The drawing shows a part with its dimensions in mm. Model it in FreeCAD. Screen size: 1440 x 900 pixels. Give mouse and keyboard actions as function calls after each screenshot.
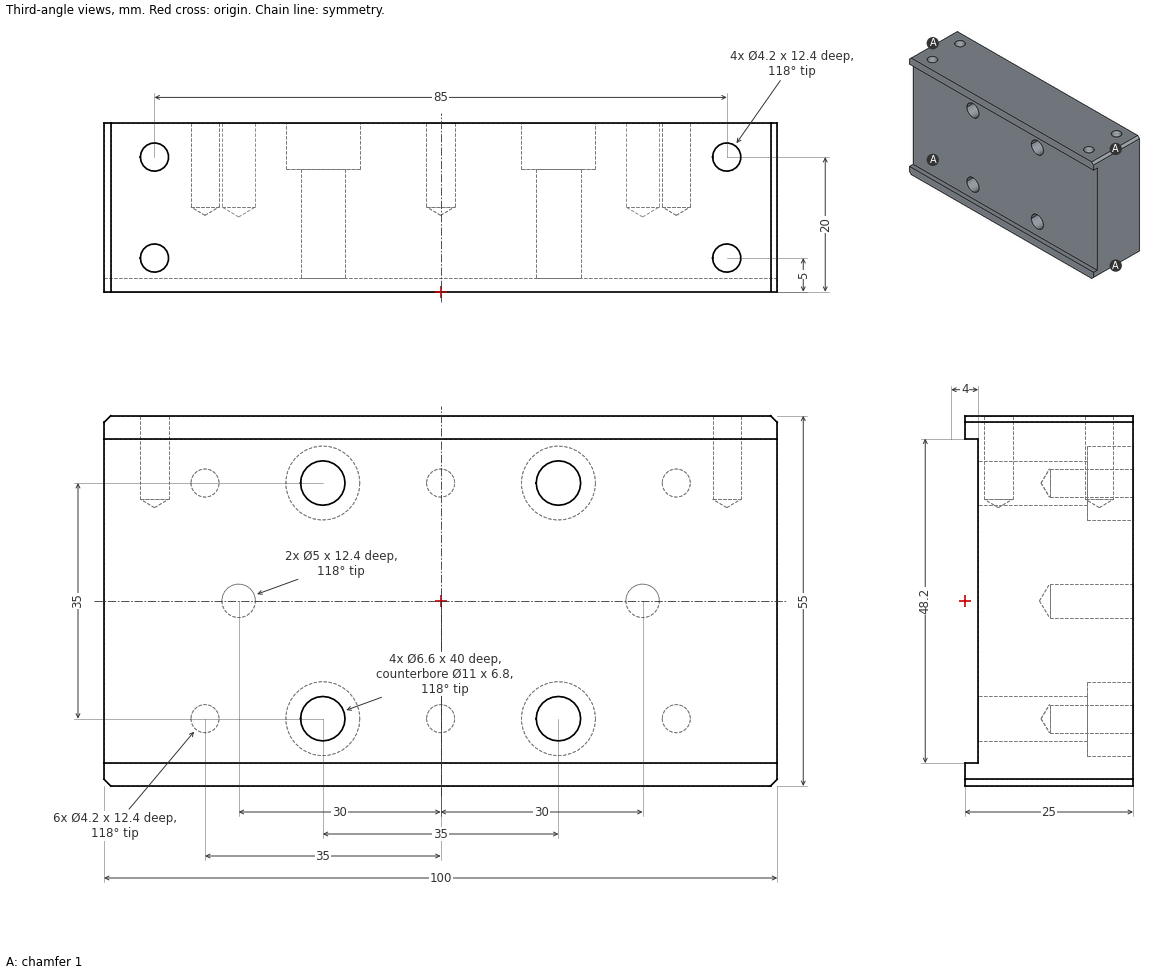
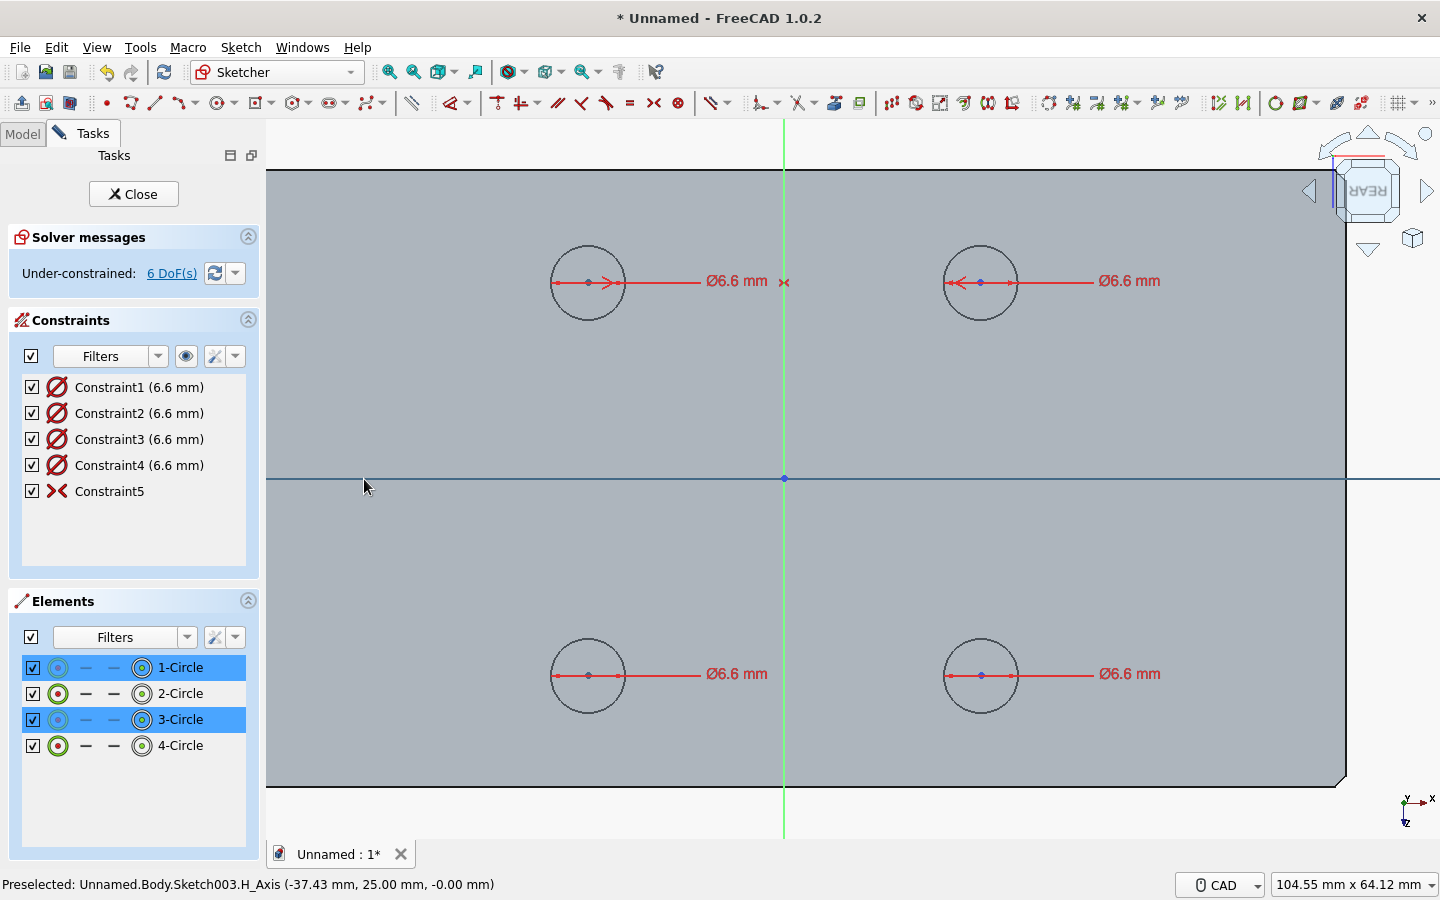
click(654, 104)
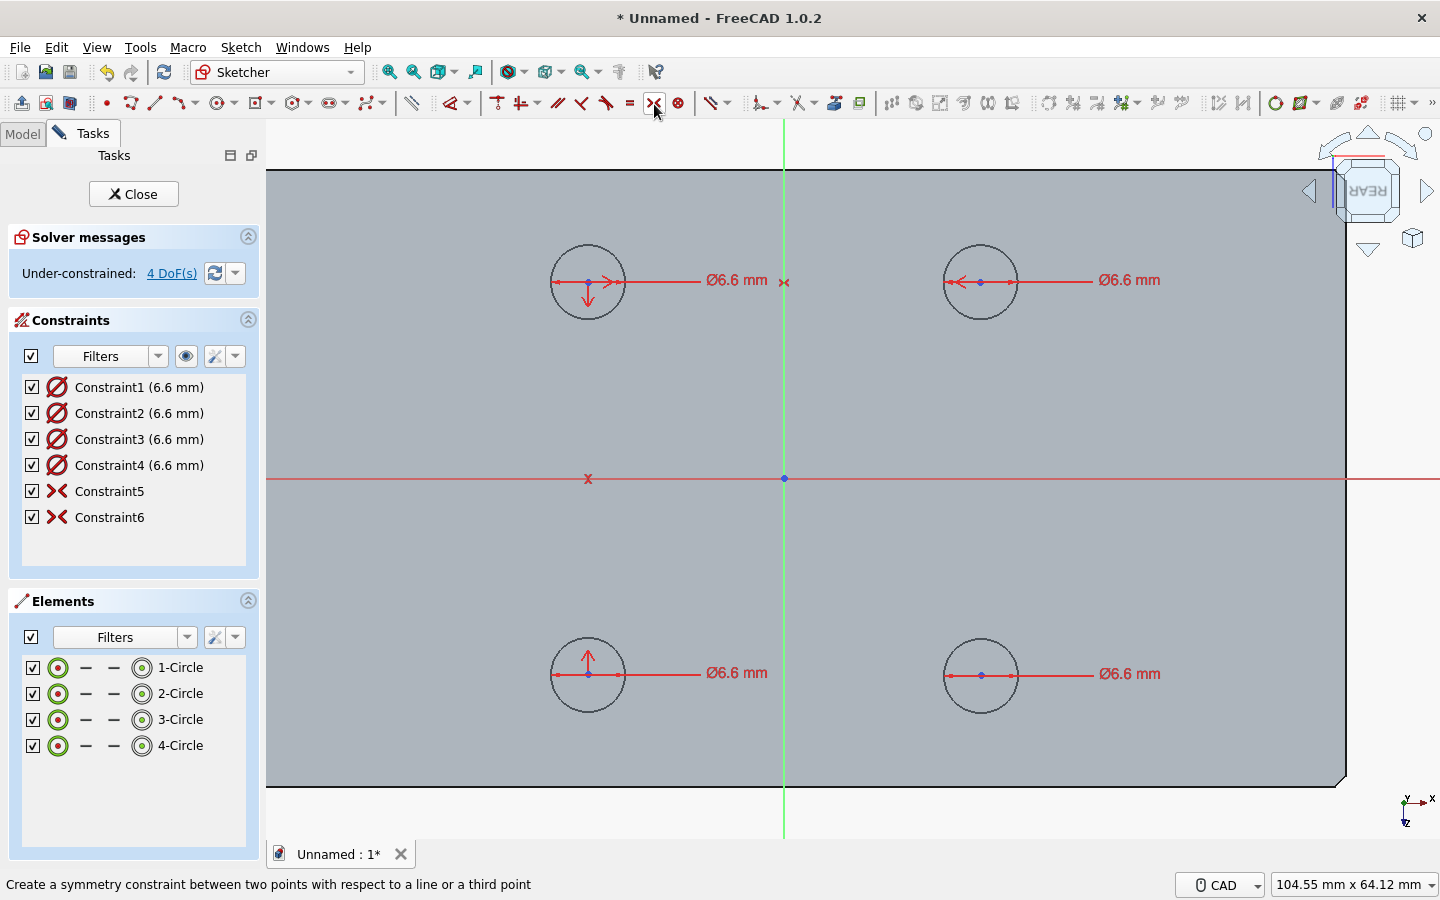
click(981, 282)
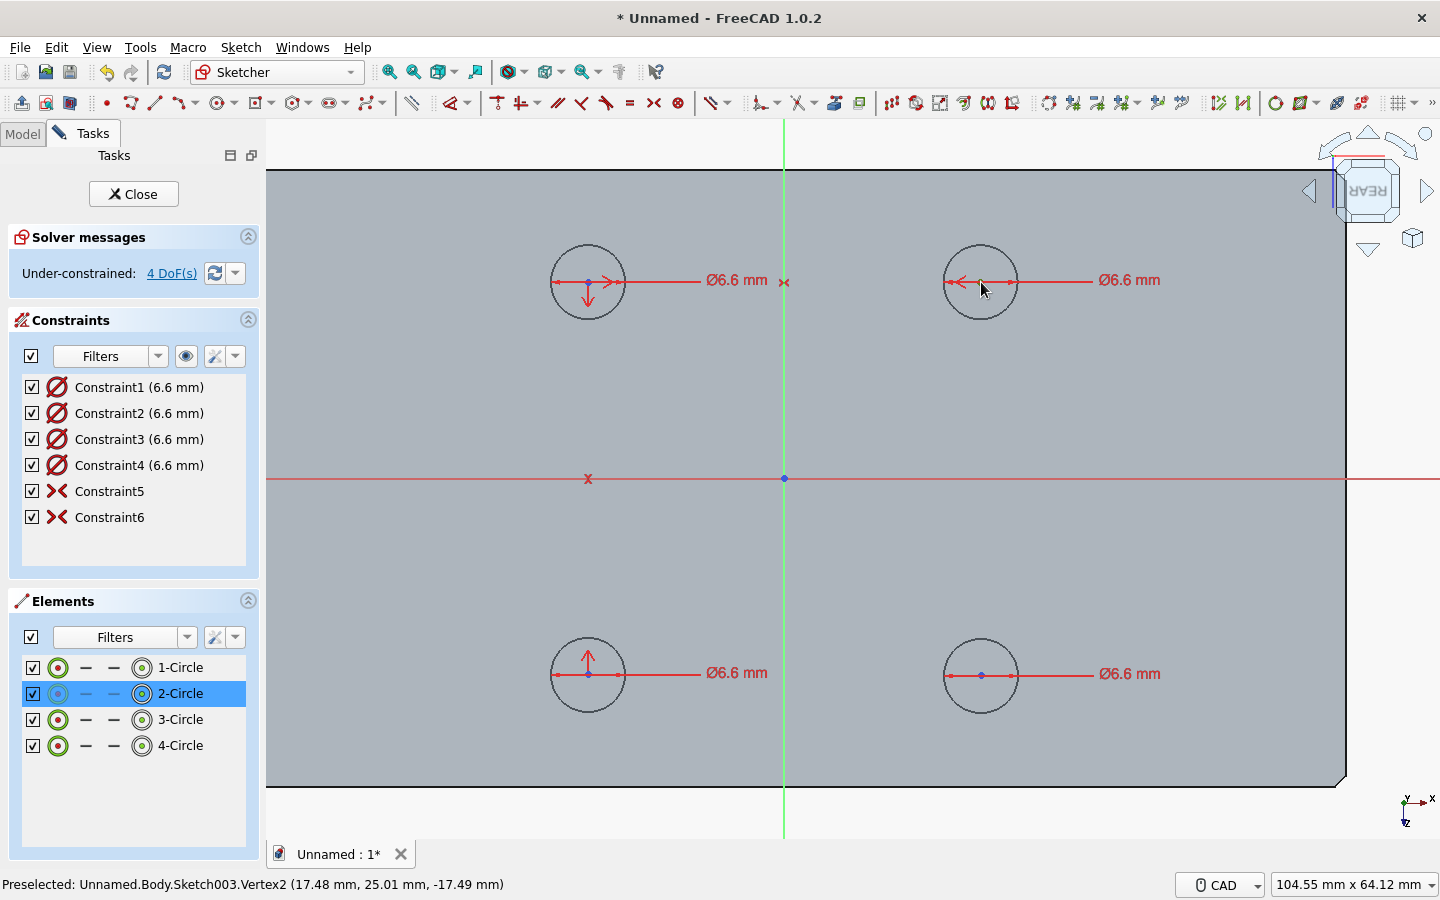
click(981, 676)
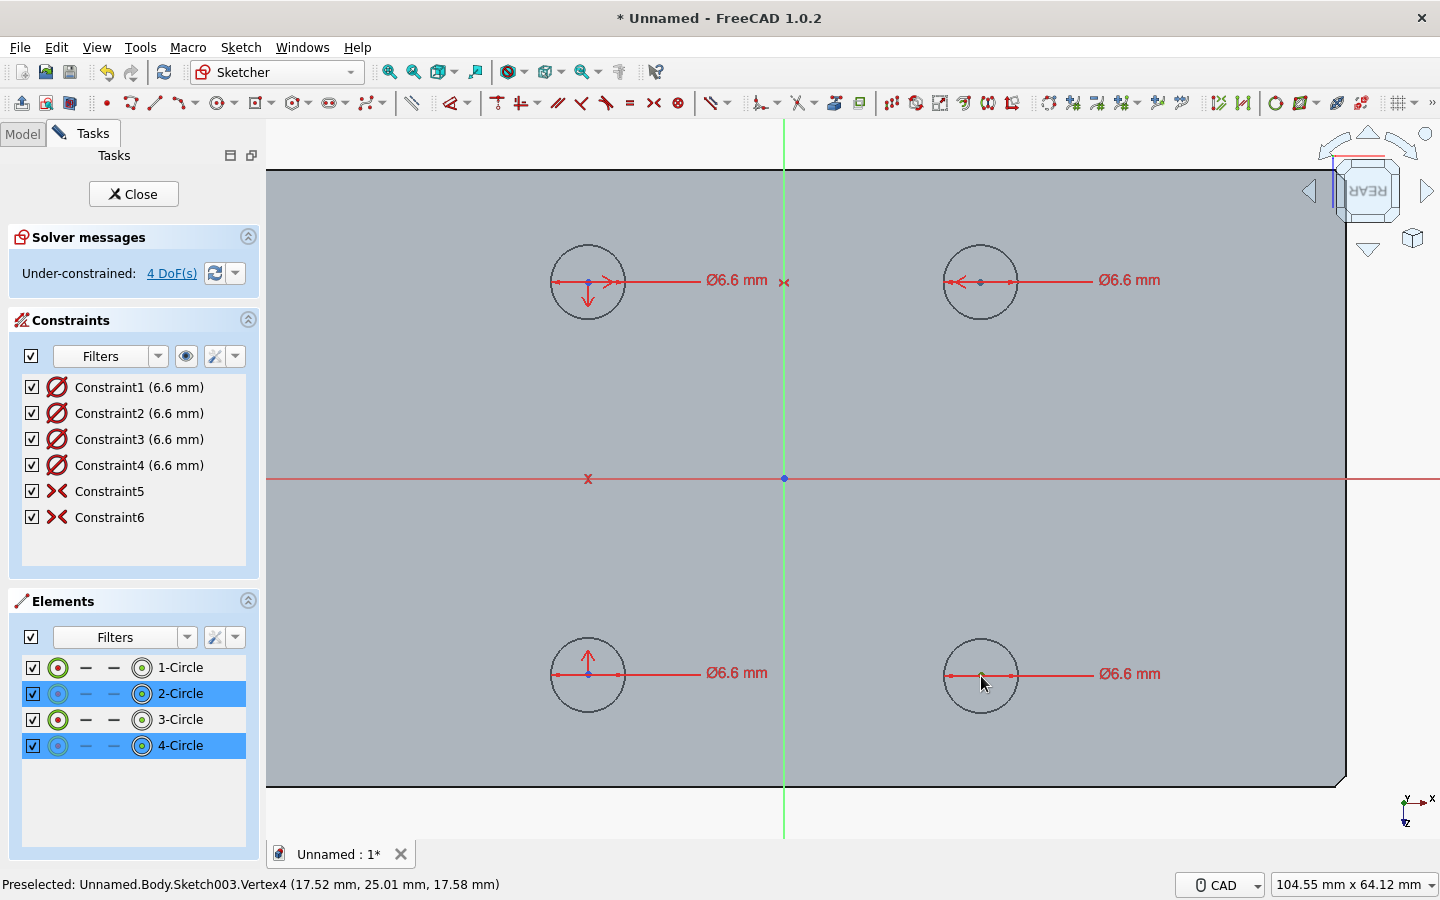
click(364, 479)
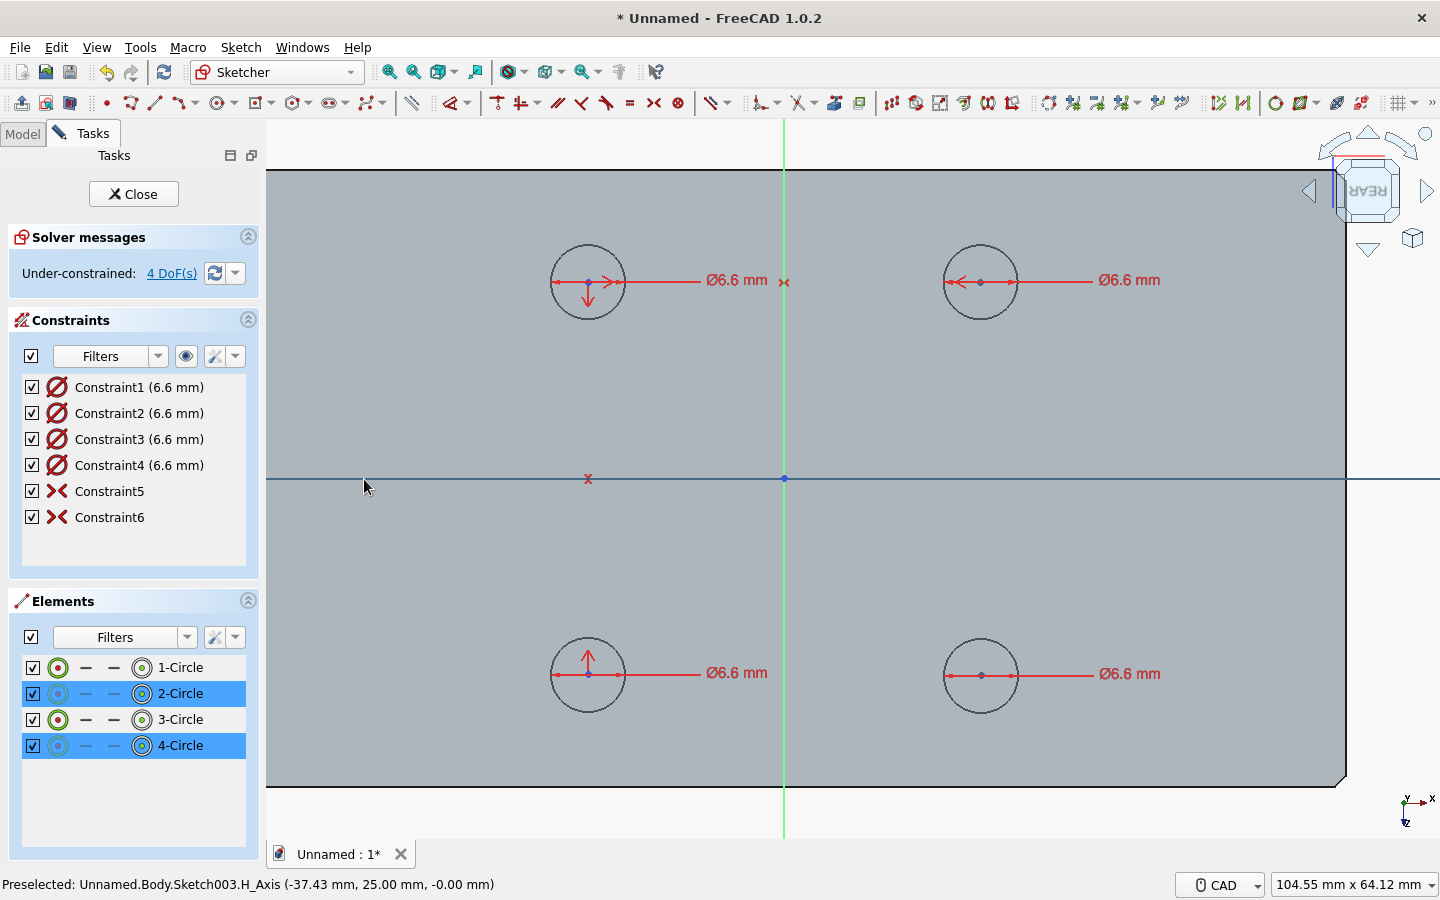
click(654, 104)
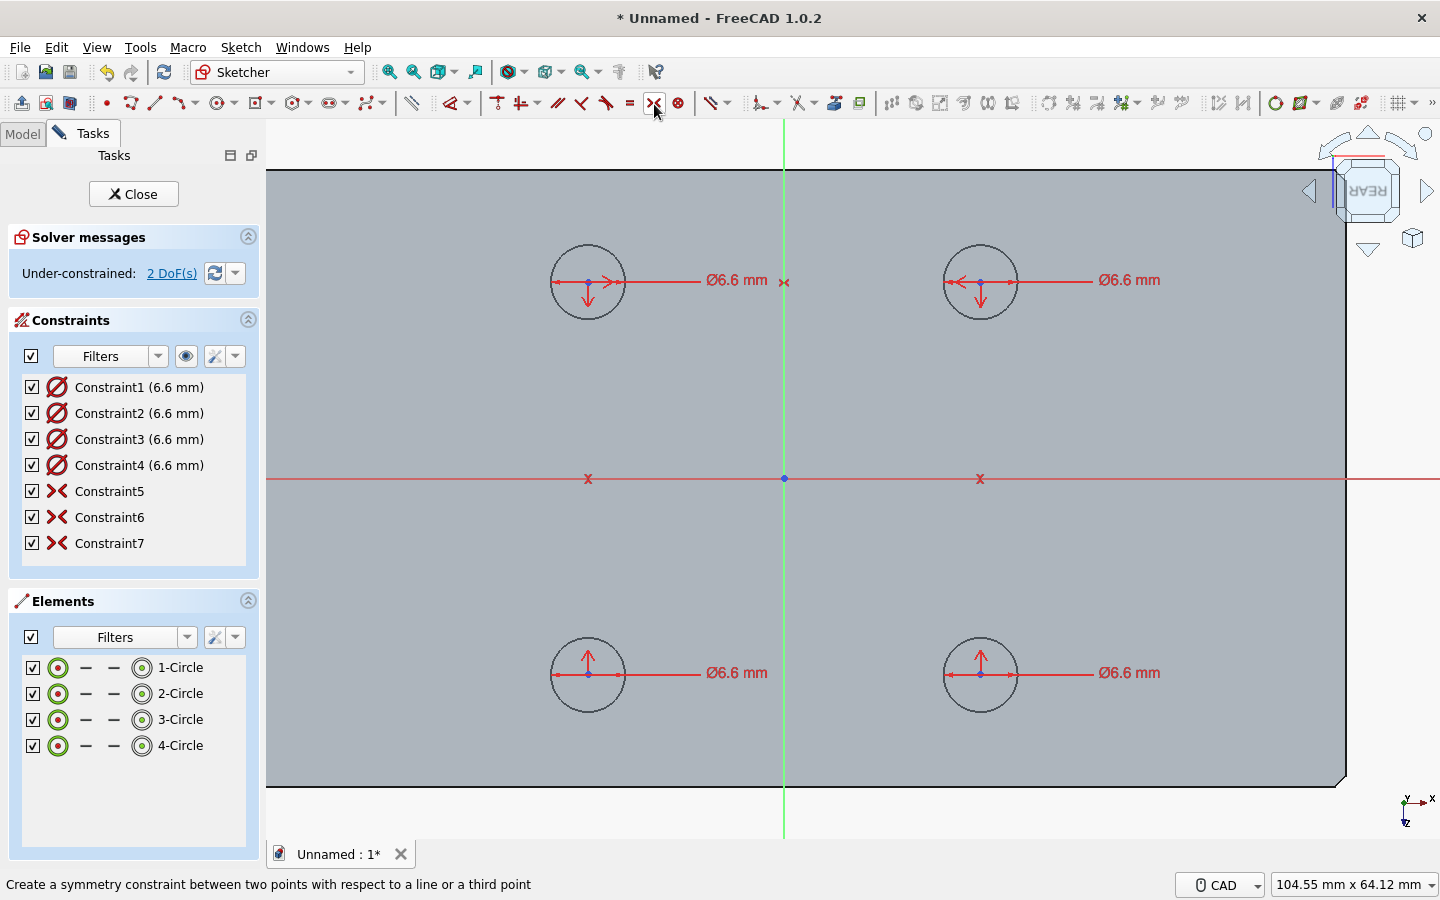
click(450, 104)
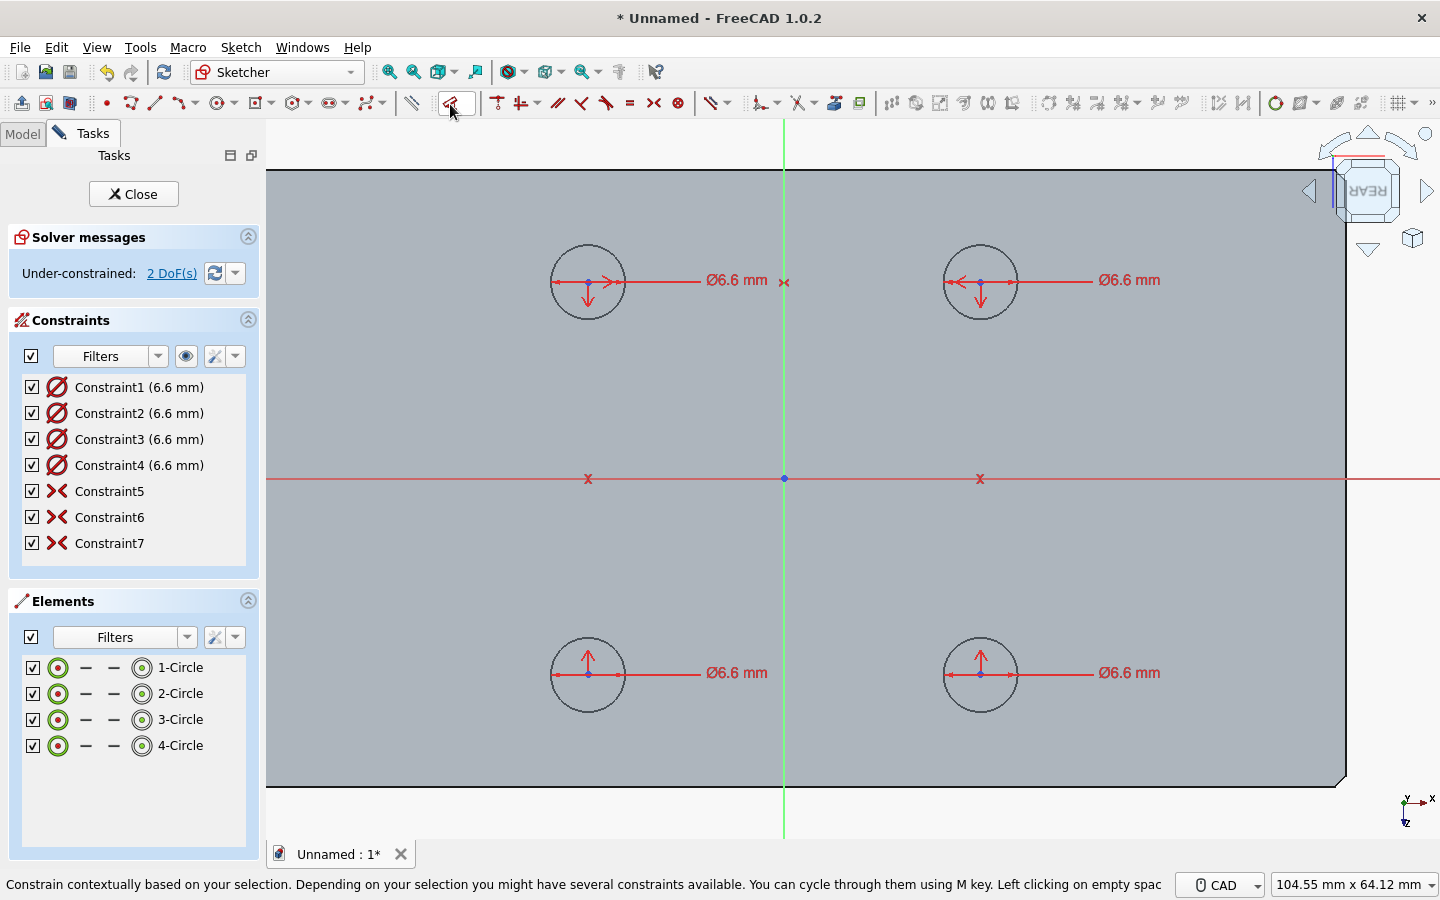
click(588, 282)